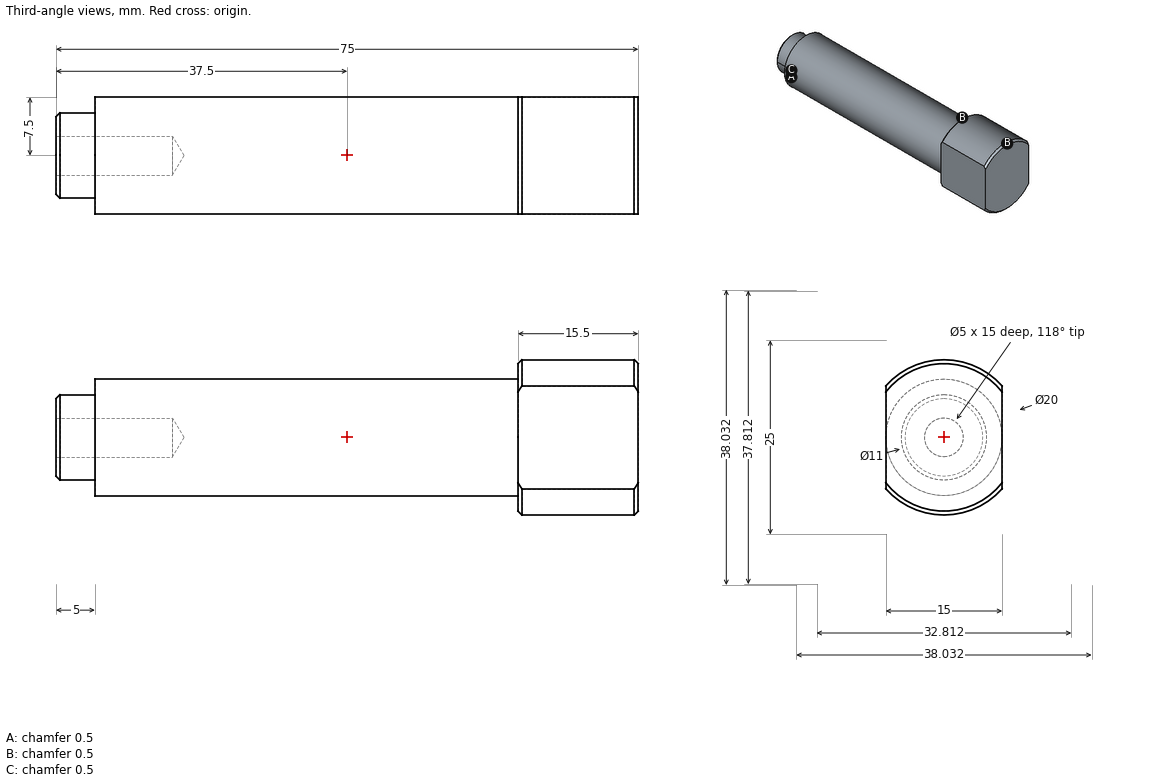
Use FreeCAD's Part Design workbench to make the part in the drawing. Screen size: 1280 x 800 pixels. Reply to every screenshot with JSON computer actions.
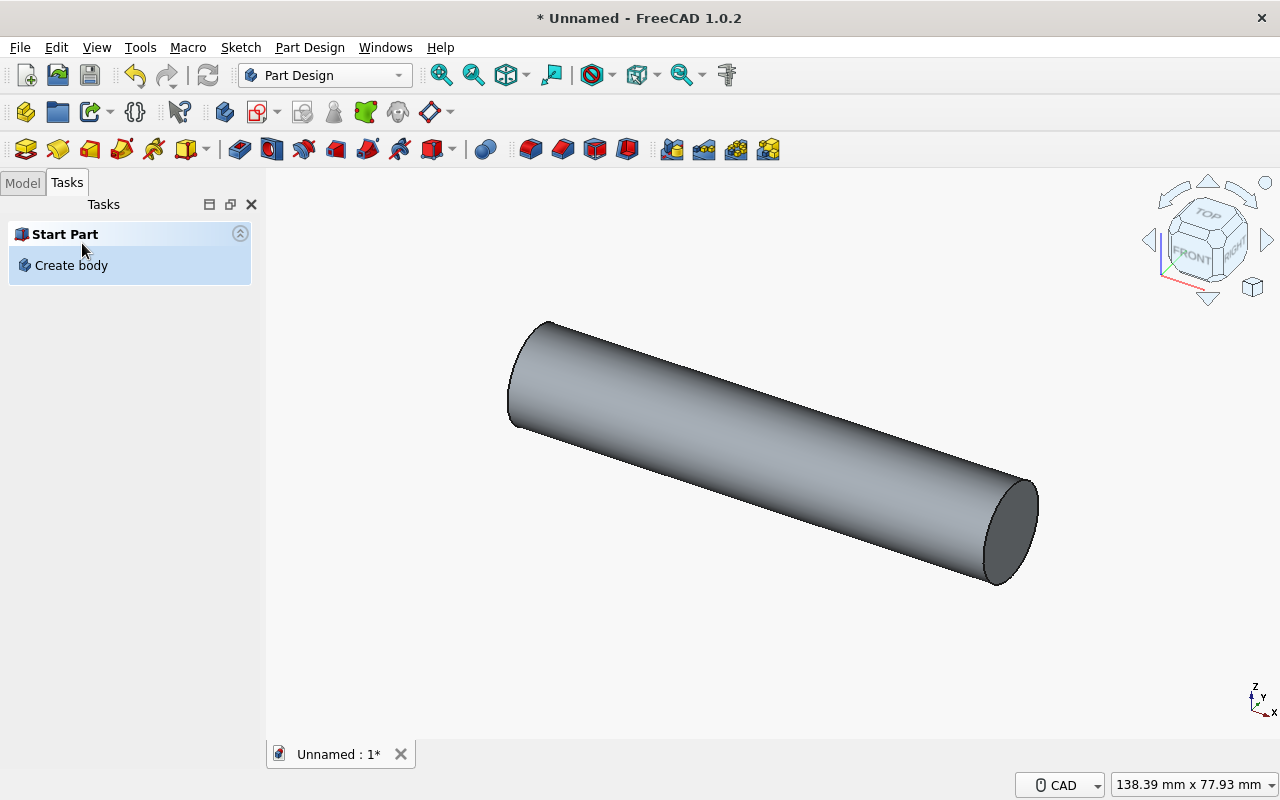
{"action": "key", "text": "0"}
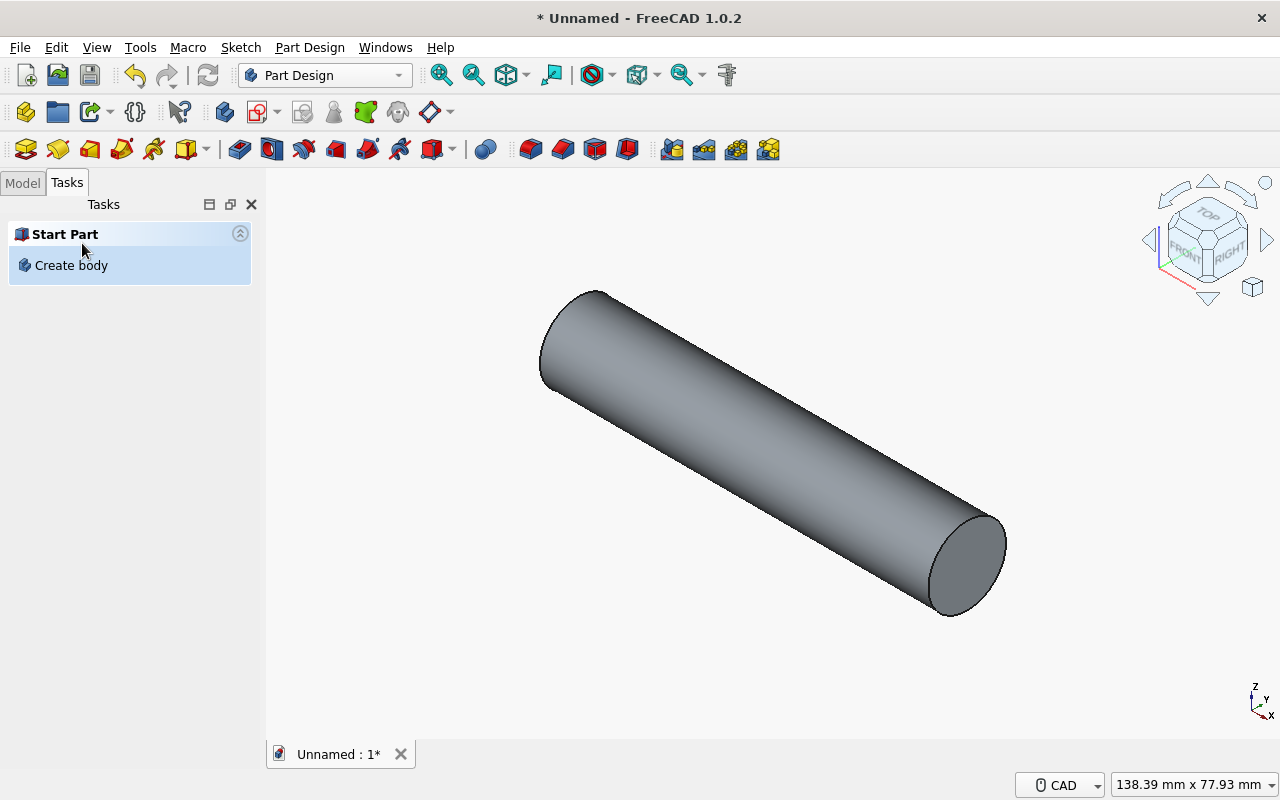
{"action": "key", "text": "2"}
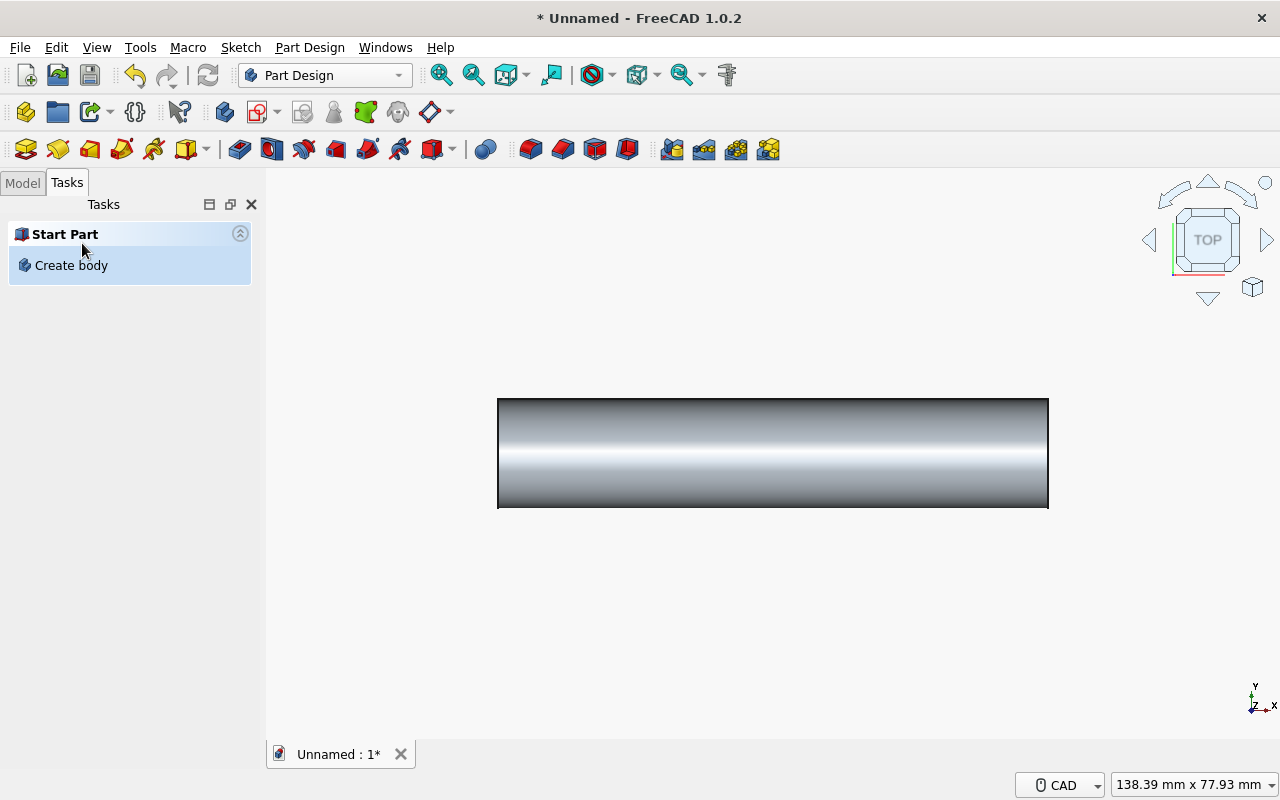
{"action": "left_click", "coordinate": [498, 497]}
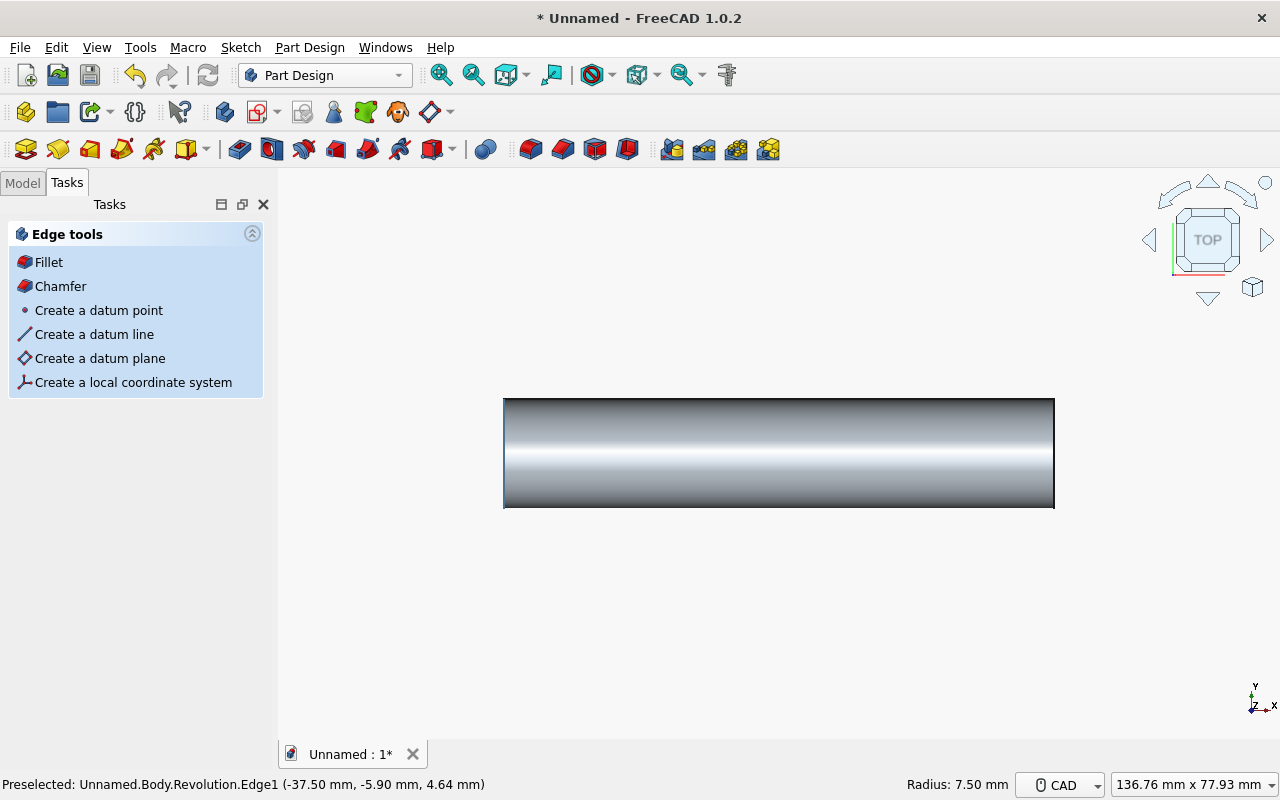
{"action": "left_click", "coordinate": [564, 150]}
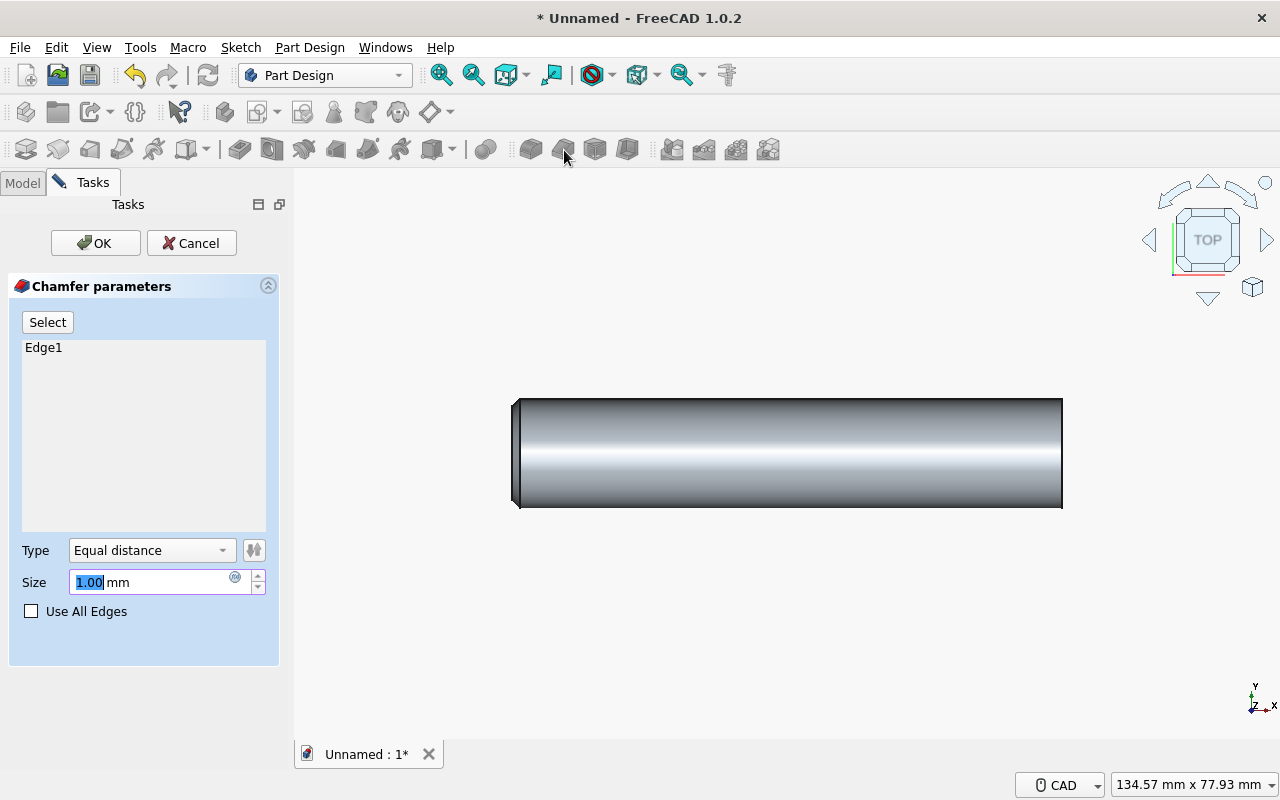
{"action": "type", "text": "0.5"}
{"action": "key", "text": "Tab"}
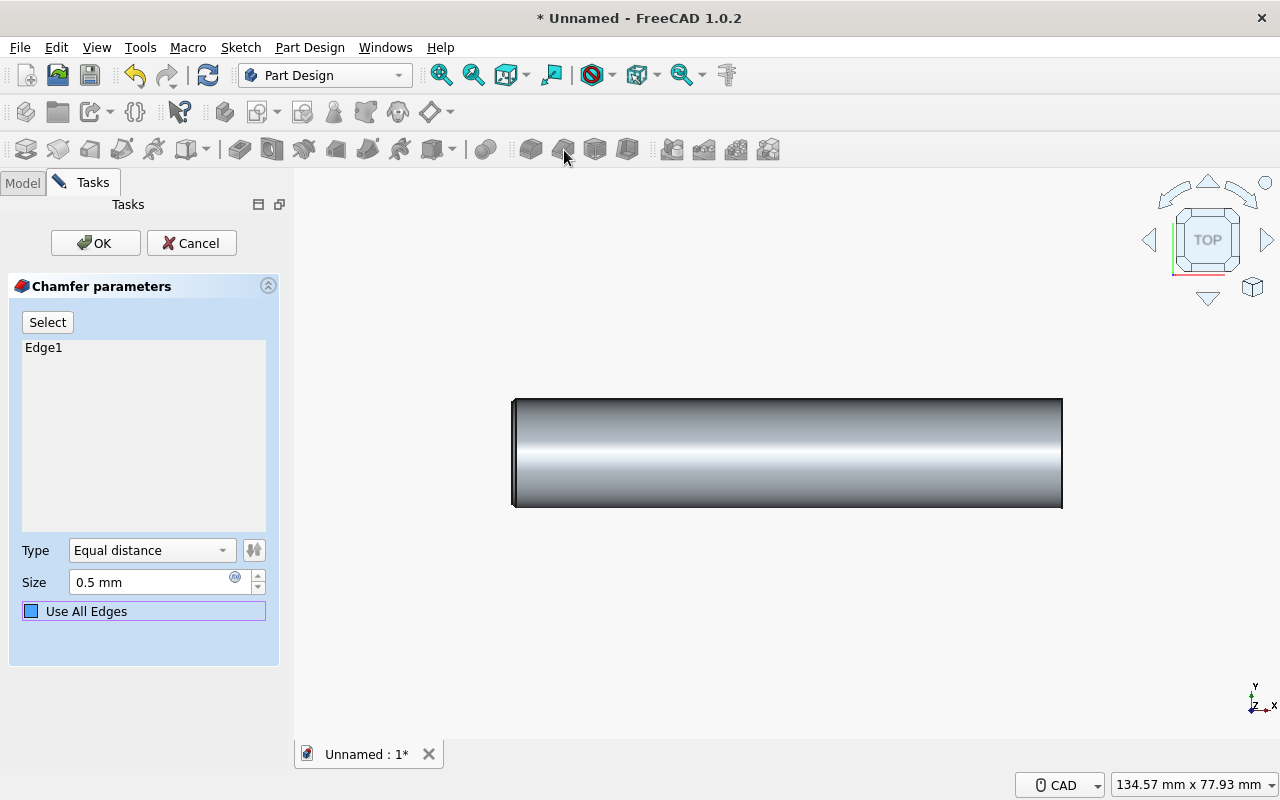
{"action": "left_click", "coordinate": [96, 243]}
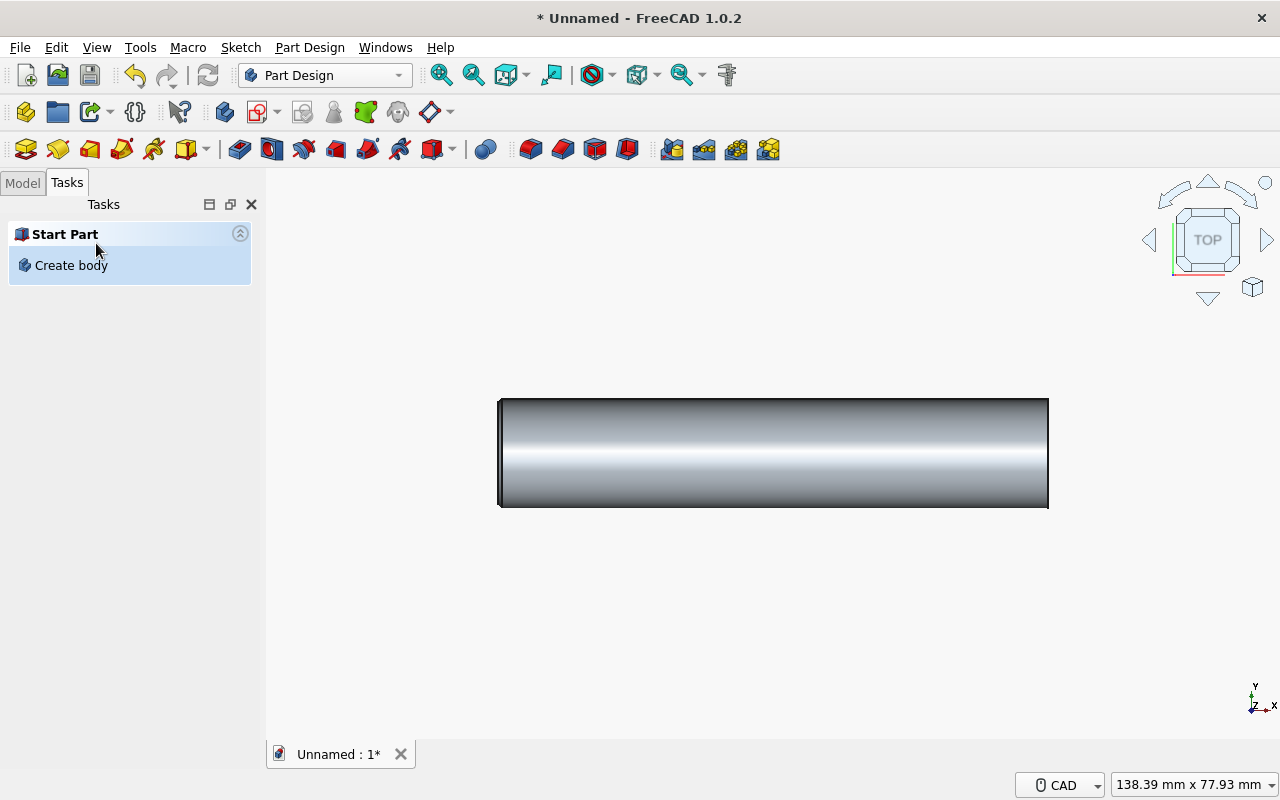
{"action": "key", "text": "6"}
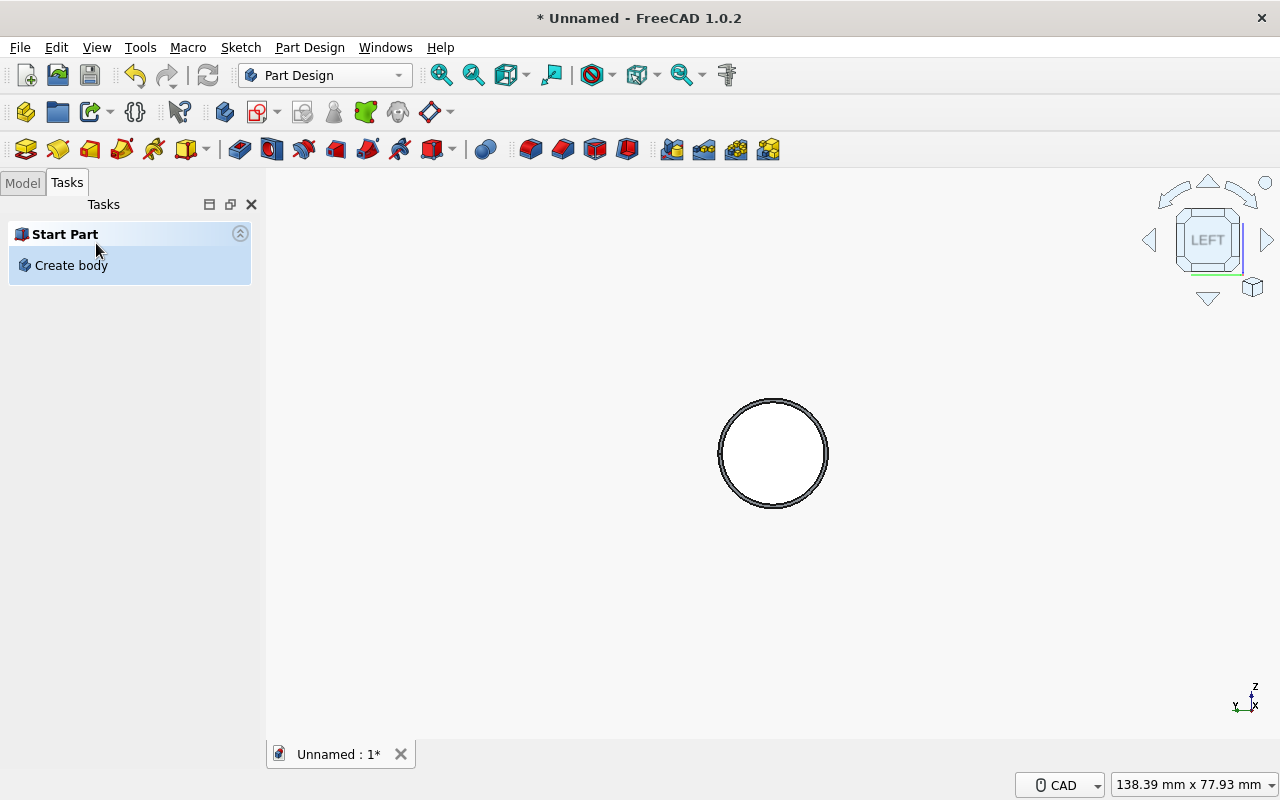
{"action": "left_click", "coordinate": [442, 76]}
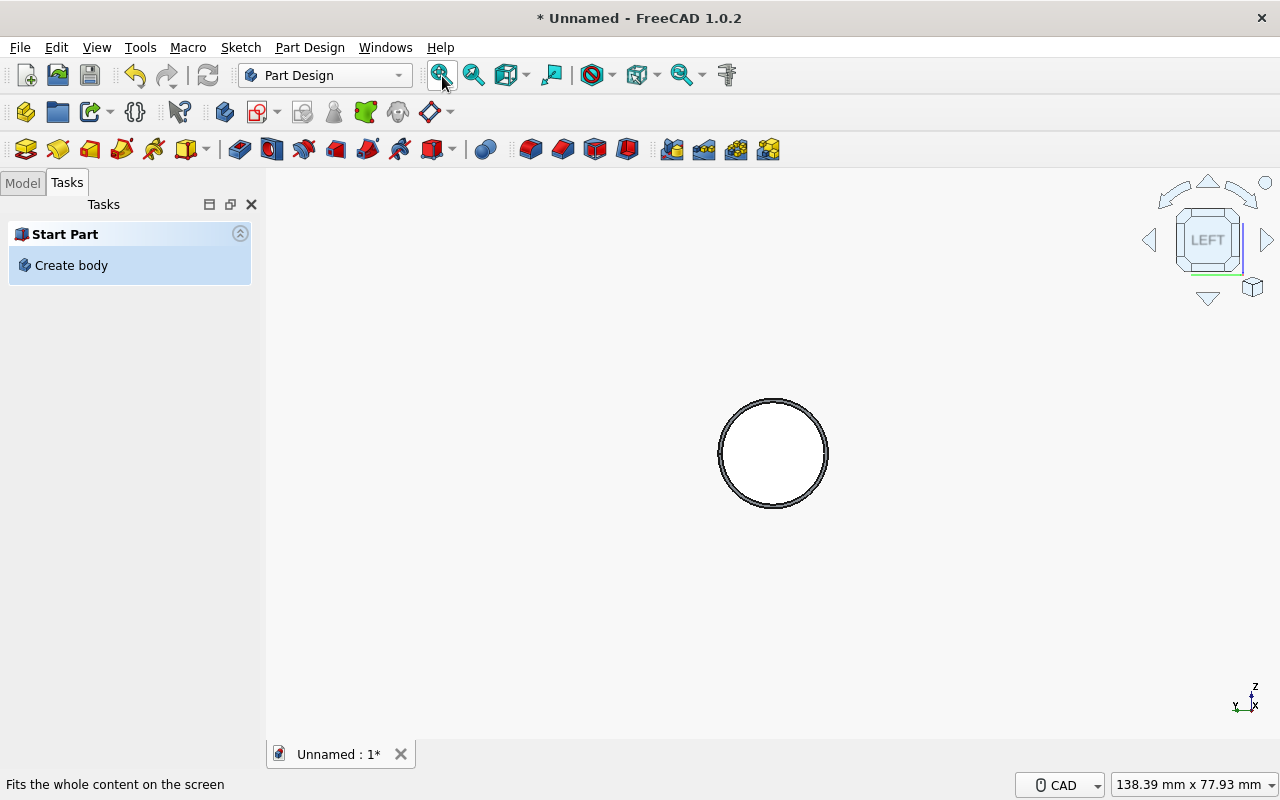
{"action": "left_click", "coordinate": [773, 452]}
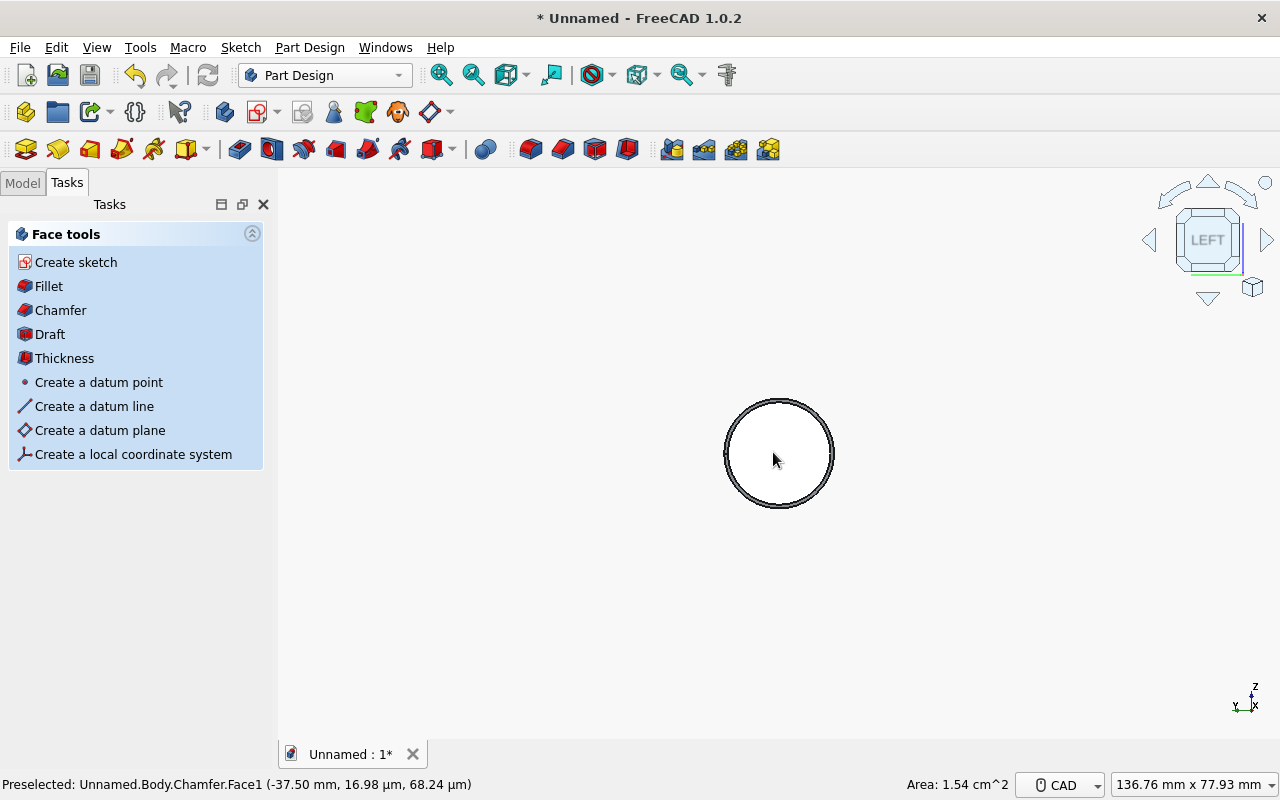
{"action": "left_click", "coordinate": [258, 112]}